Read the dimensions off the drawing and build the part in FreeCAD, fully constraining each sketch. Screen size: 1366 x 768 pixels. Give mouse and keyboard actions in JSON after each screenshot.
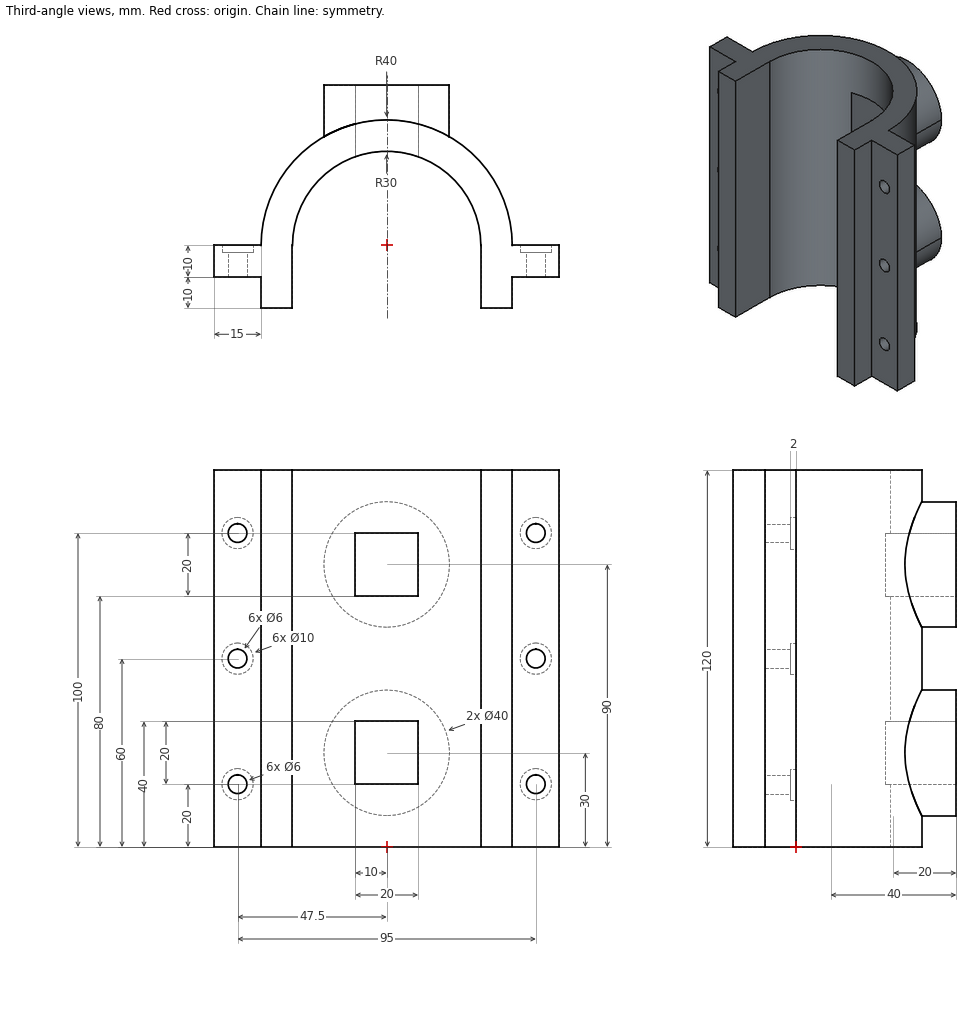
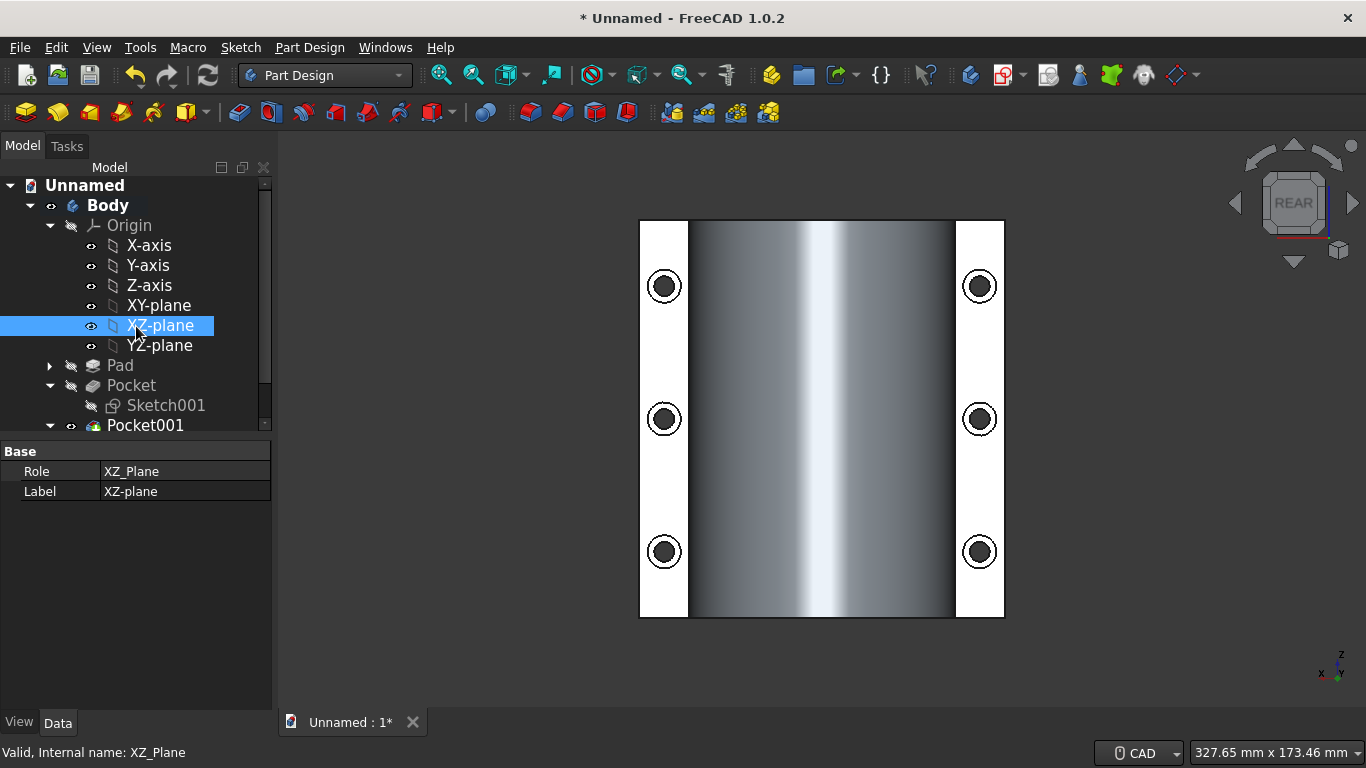
{"action": "left_click", "coordinate": [1176, 76]}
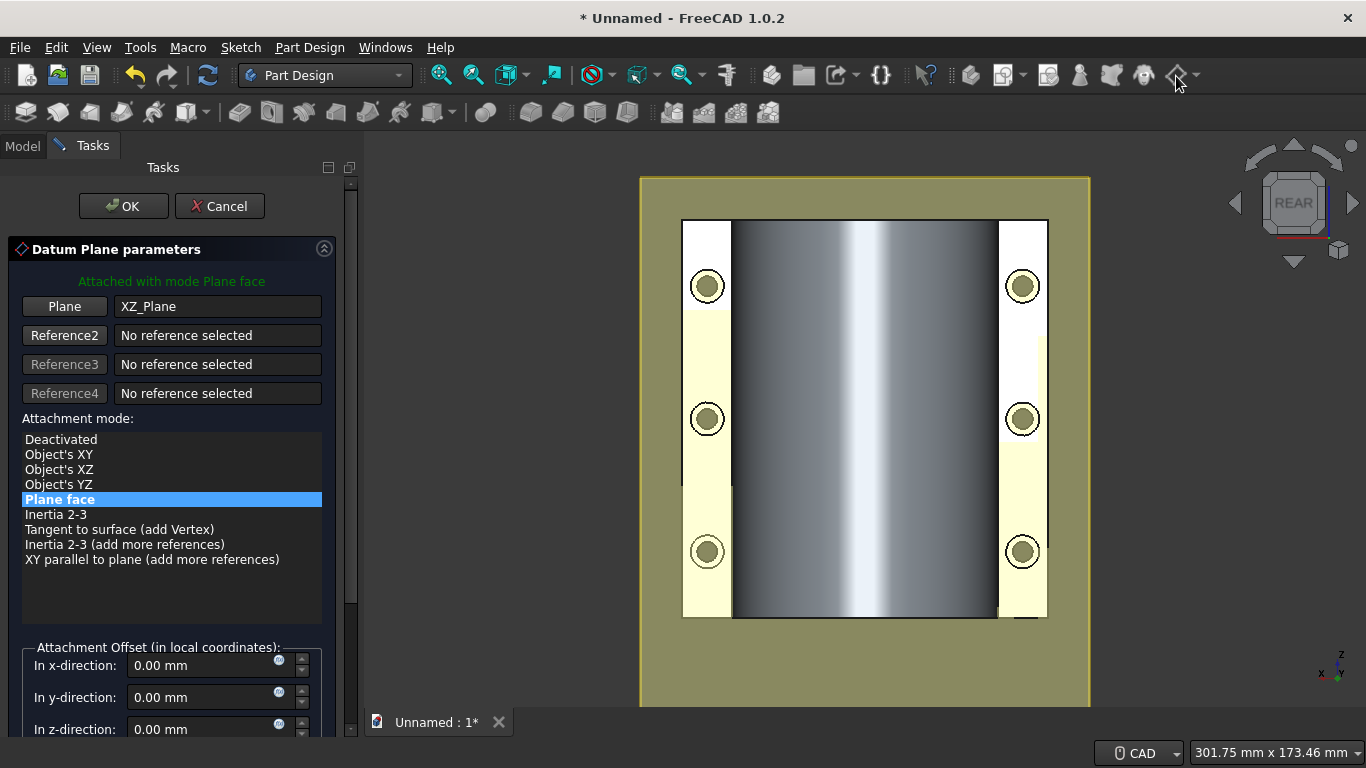
{"action": "scroll", "coordinate": [351, 456], "scroll_direction": "down", "scroll_amount": 2}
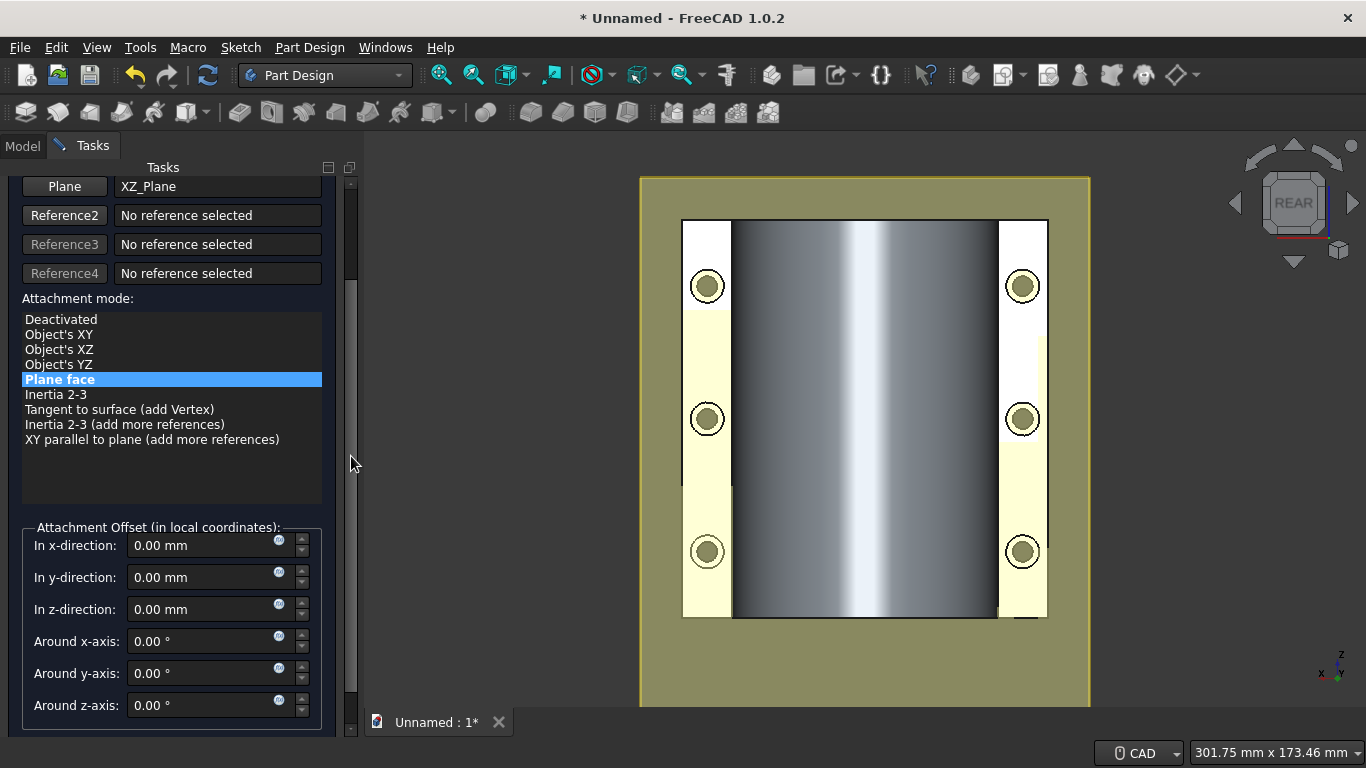
{"action": "triple_click", "coordinate": [210, 609]}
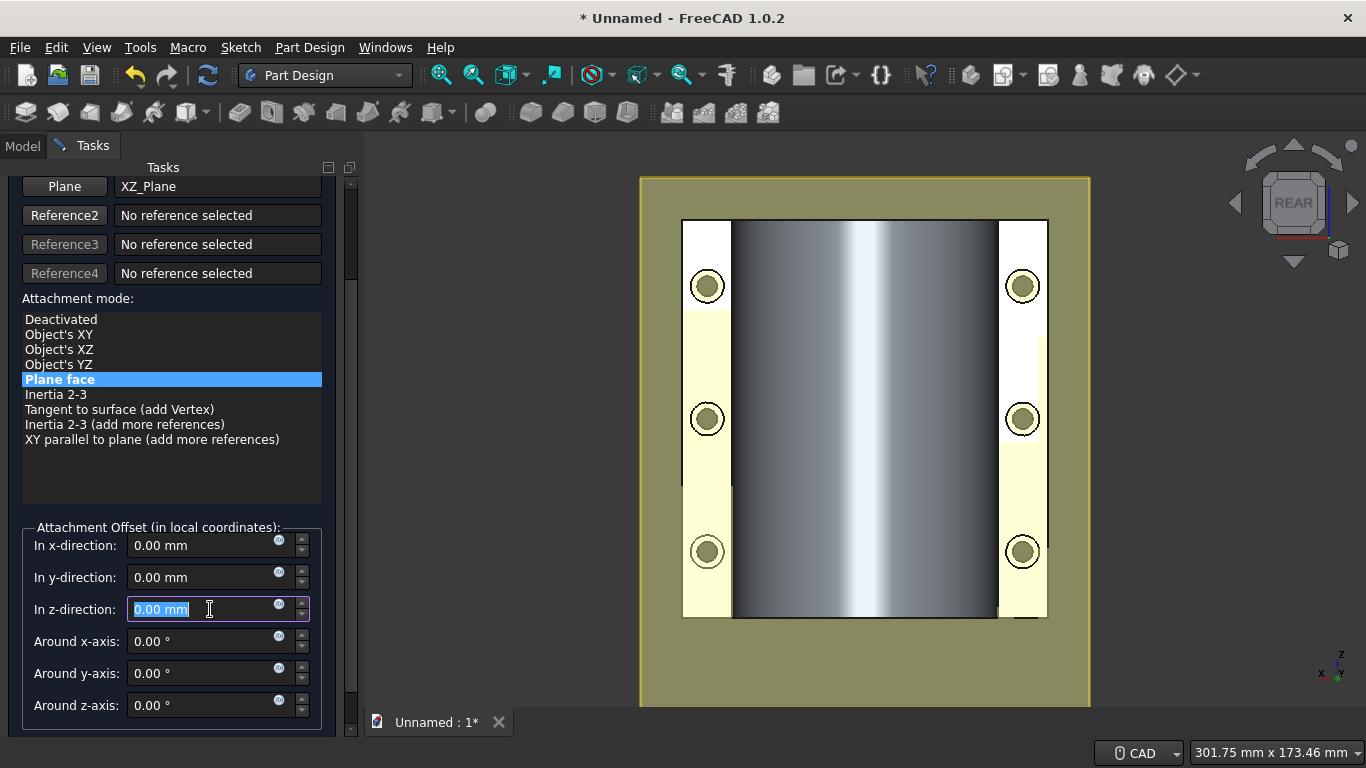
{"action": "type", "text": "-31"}
{"action": "key", "text": "Tab"}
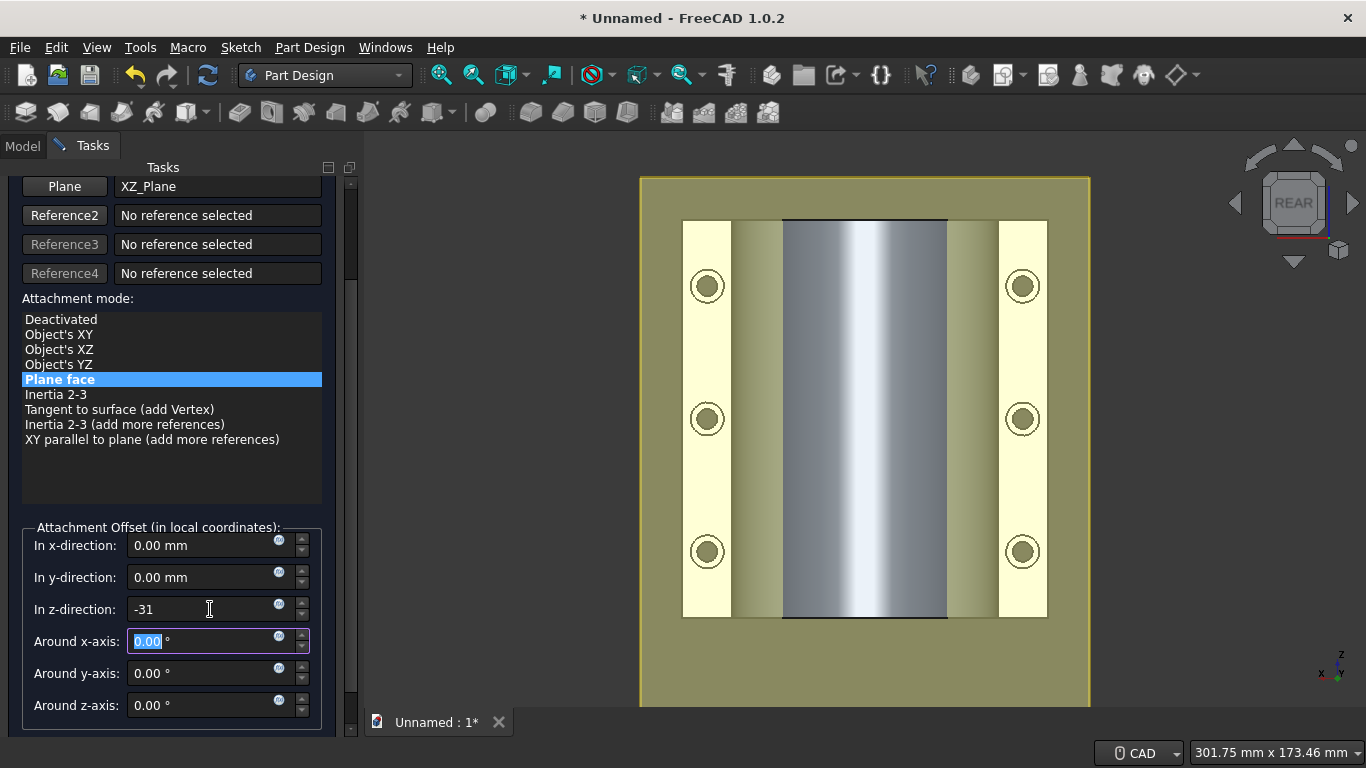
{"action": "scroll", "coordinate": [351, 456], "scroll_direction": "up", "scroll_amount": 3}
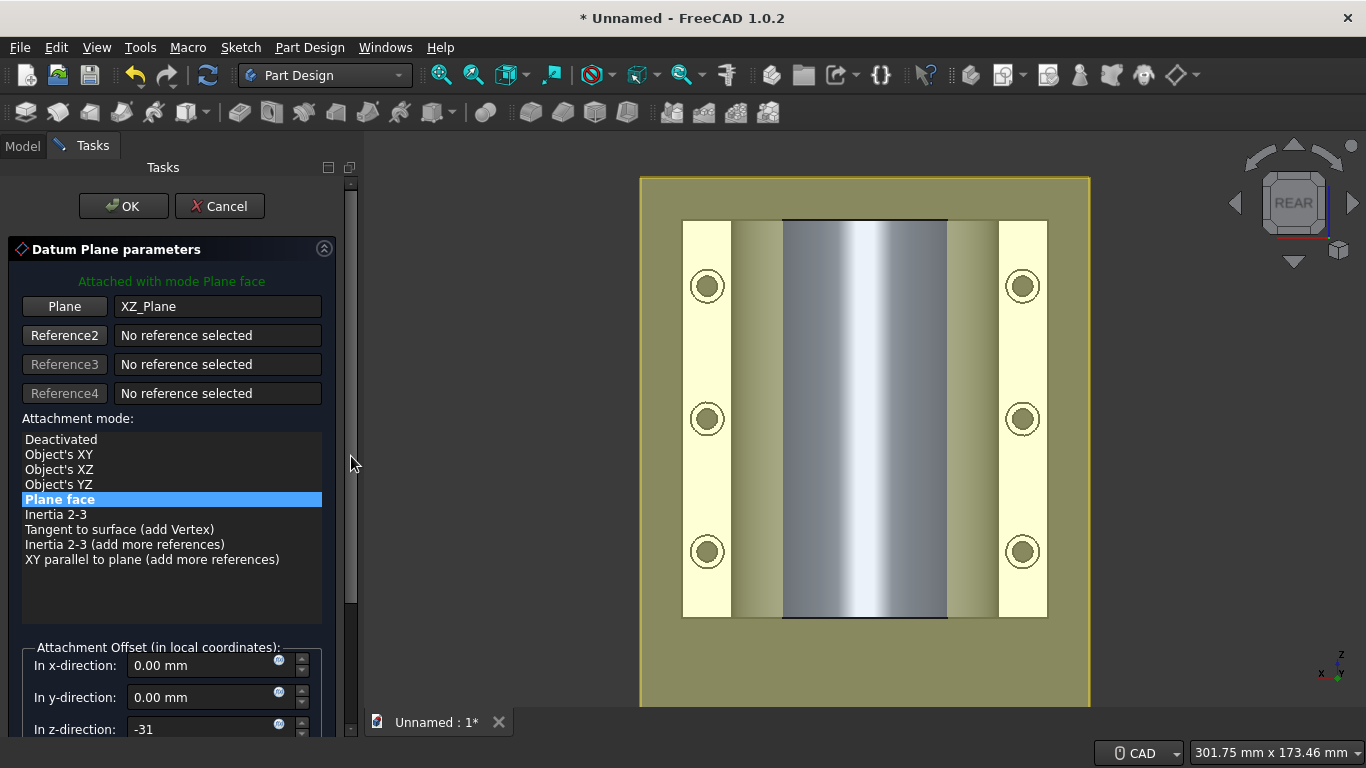
{"action": "left_click", "coordinate": [124, 206]}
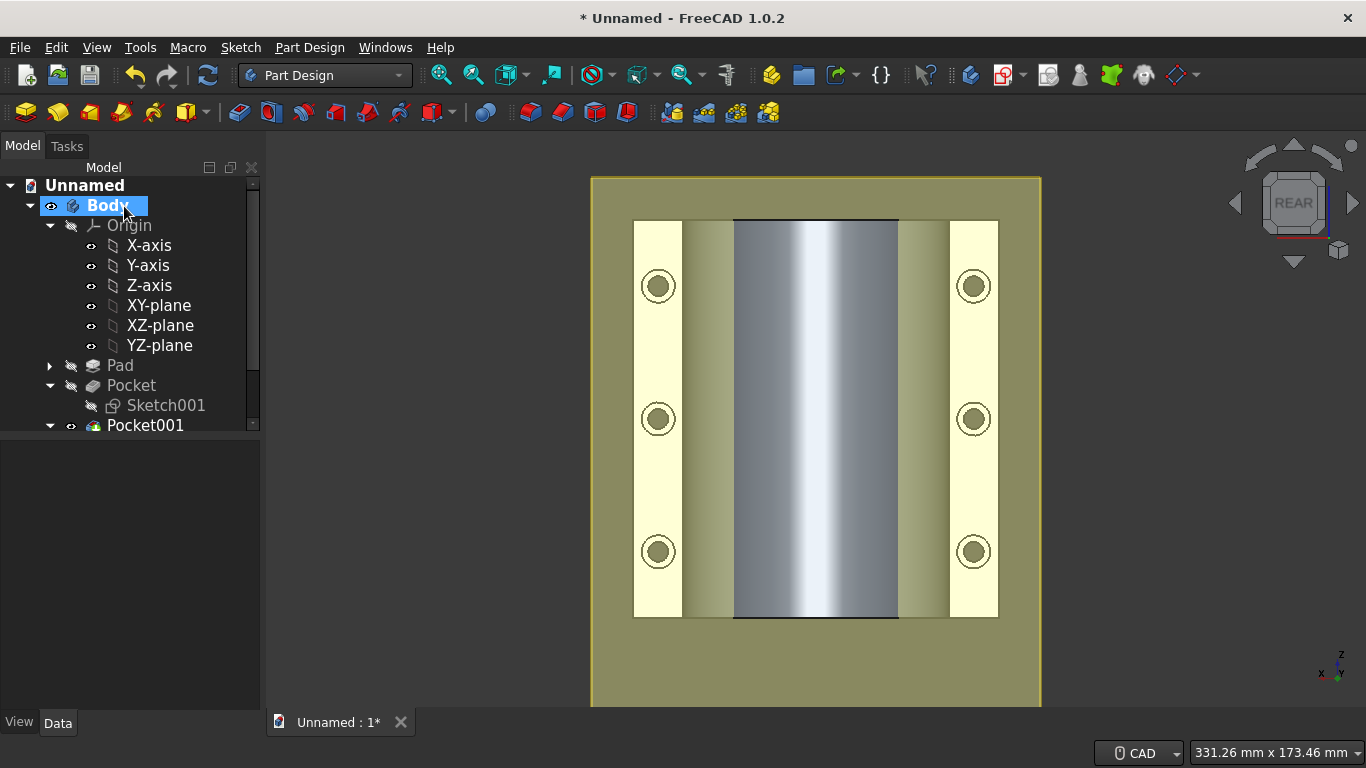
{"action": "scroll", "coordinate": [100, 301], "scroll_direction": "down", "scroll_amount": 3}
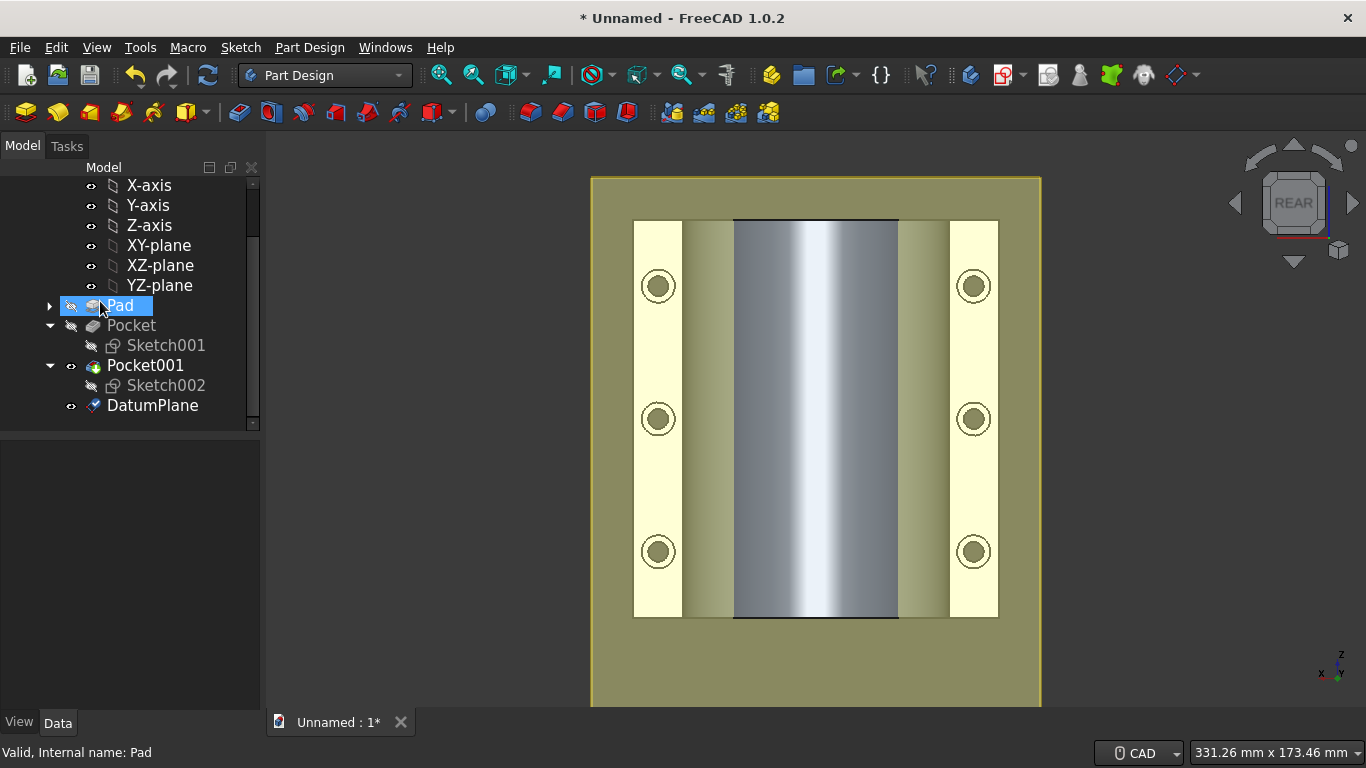
{"action": "left_click", "coordinate": [116, 406]}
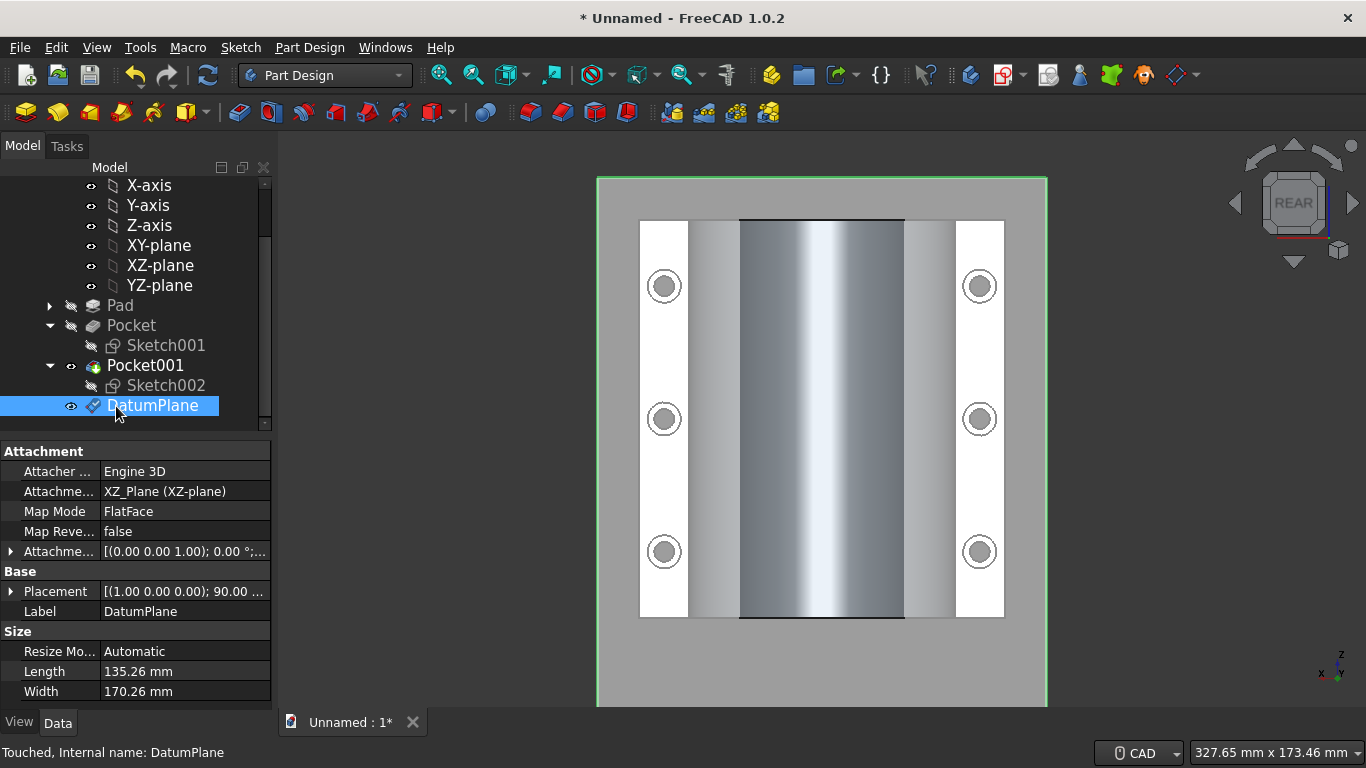
{"action": "left_click", "coordinate": [1004, 76]}